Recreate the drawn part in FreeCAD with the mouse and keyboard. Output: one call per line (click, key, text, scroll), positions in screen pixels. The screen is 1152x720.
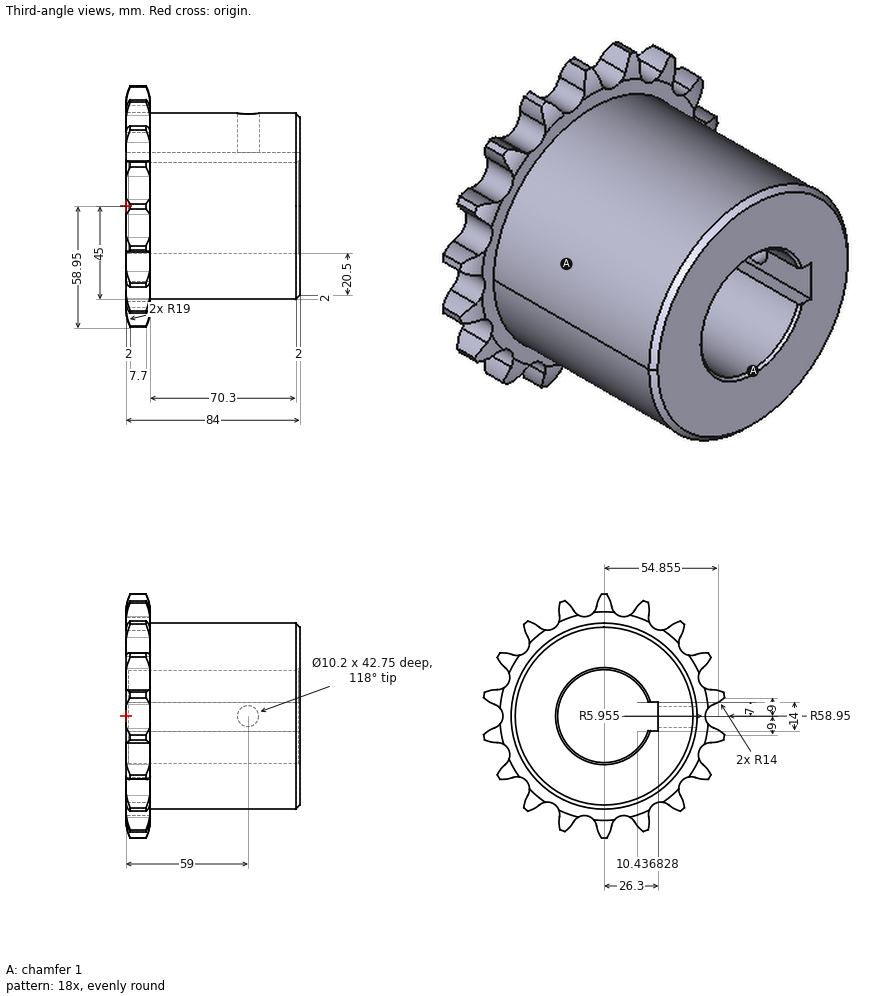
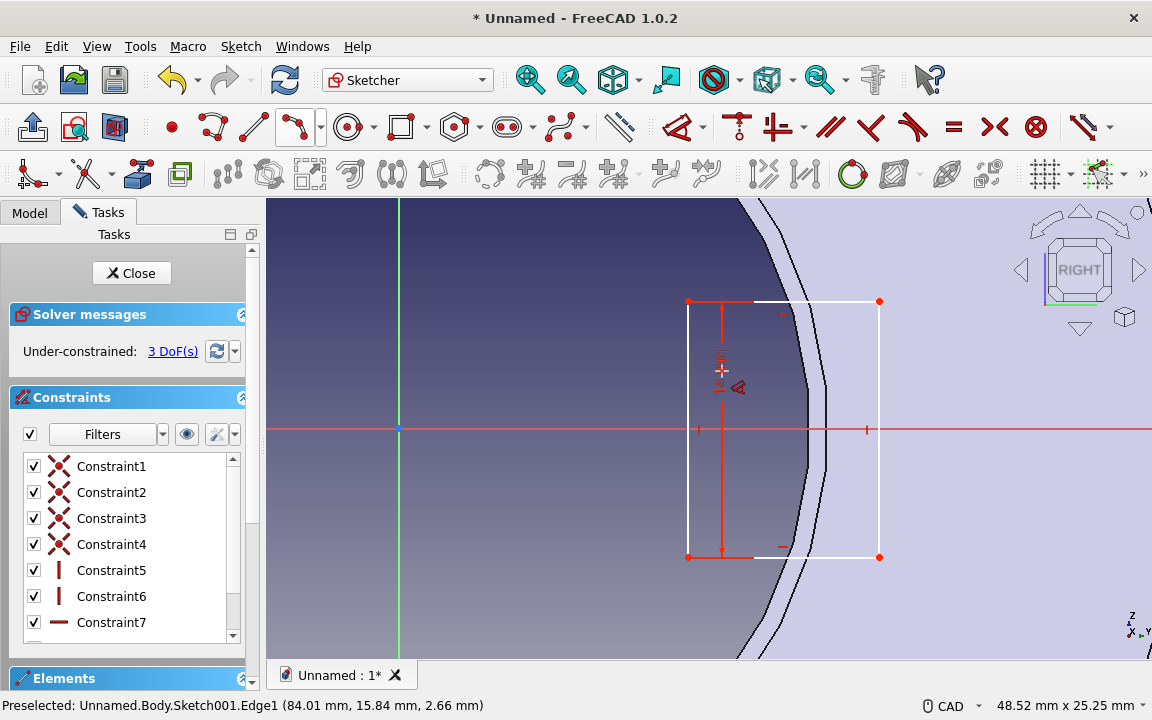
click(688, 302)
click(365, 365)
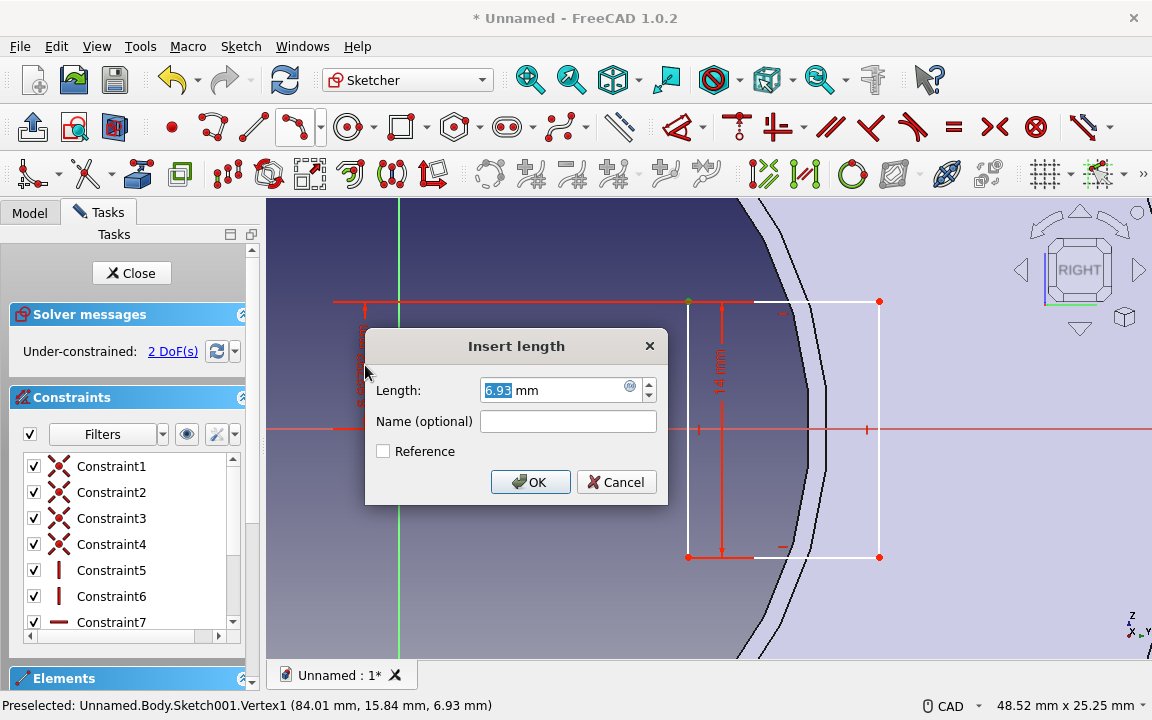
text(7)
key(Return)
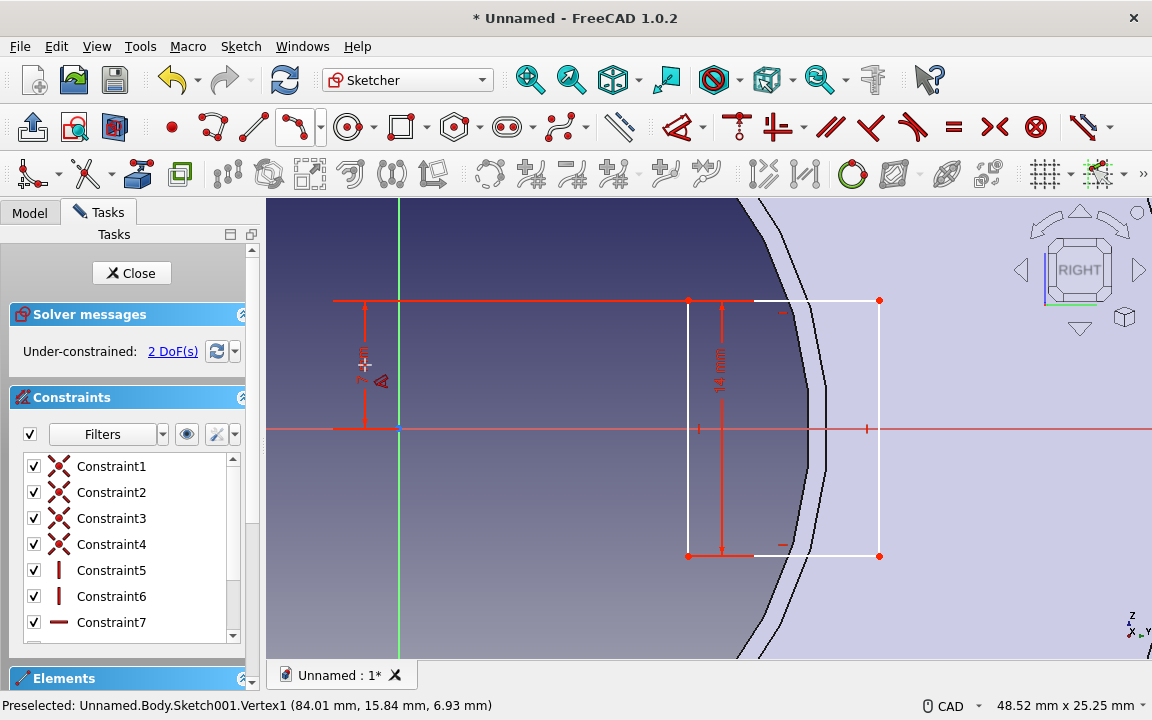
click(879, 556)
click(639, 590)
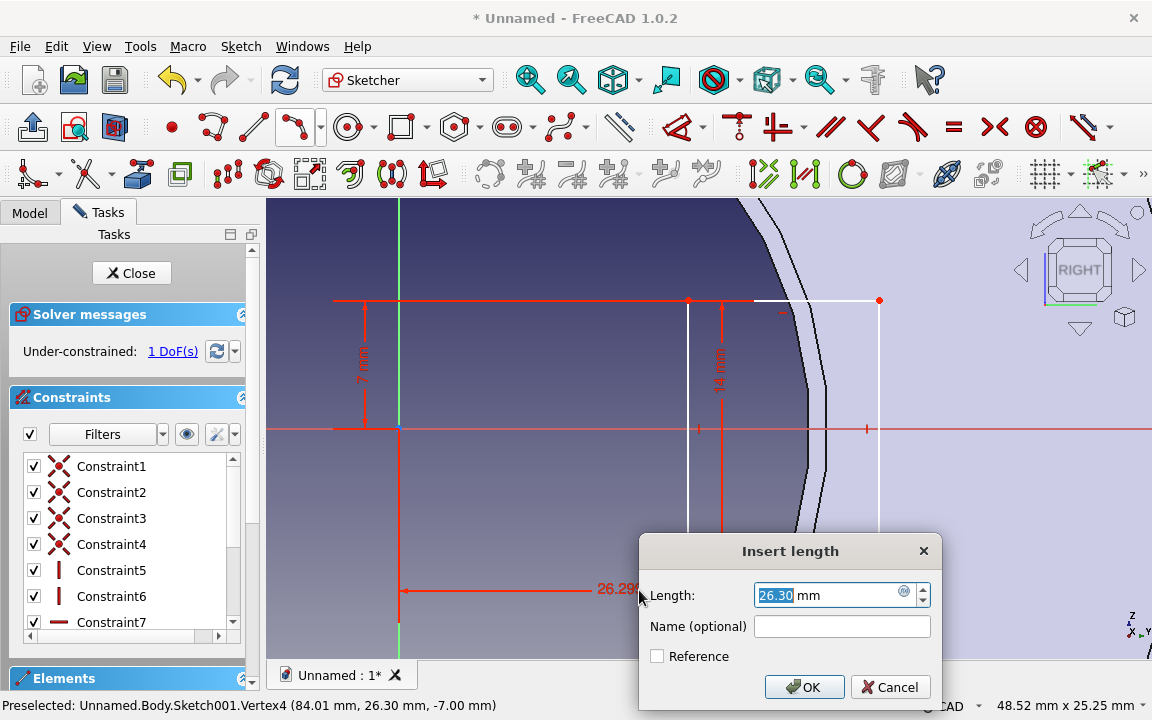
text(26.3)
key(Return)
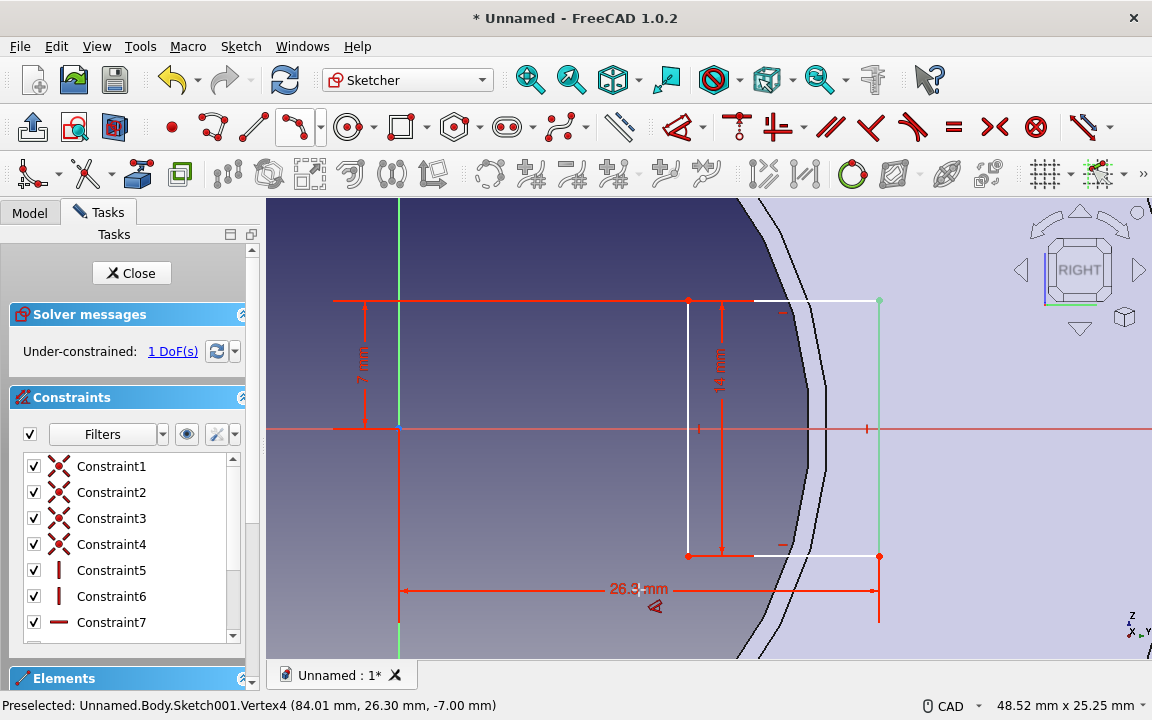
click(745, 556)
click(784, 590)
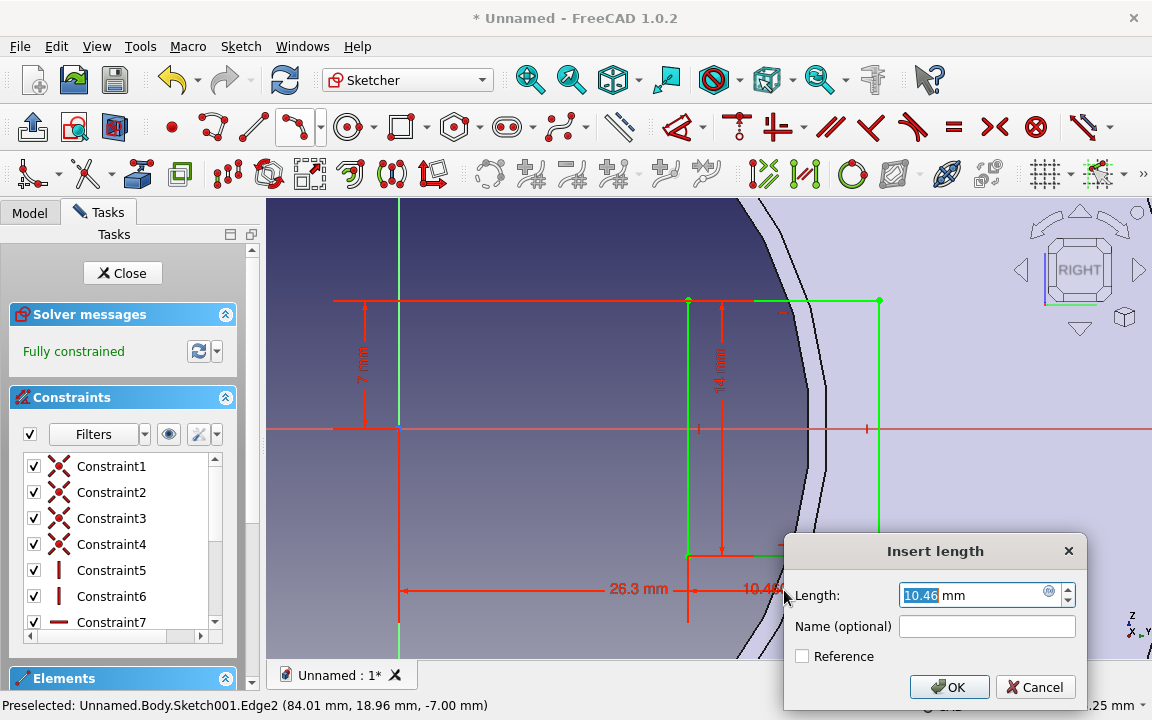
text(10.436828)
key(Return)
key(Escape)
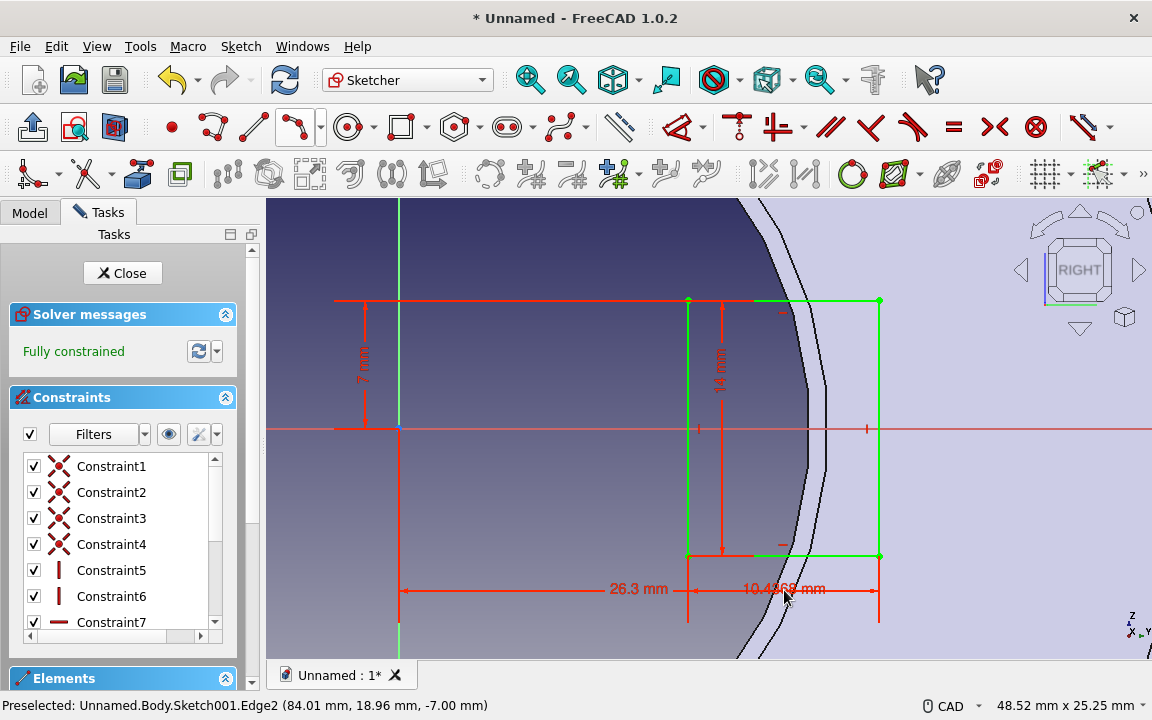
click(123, 273)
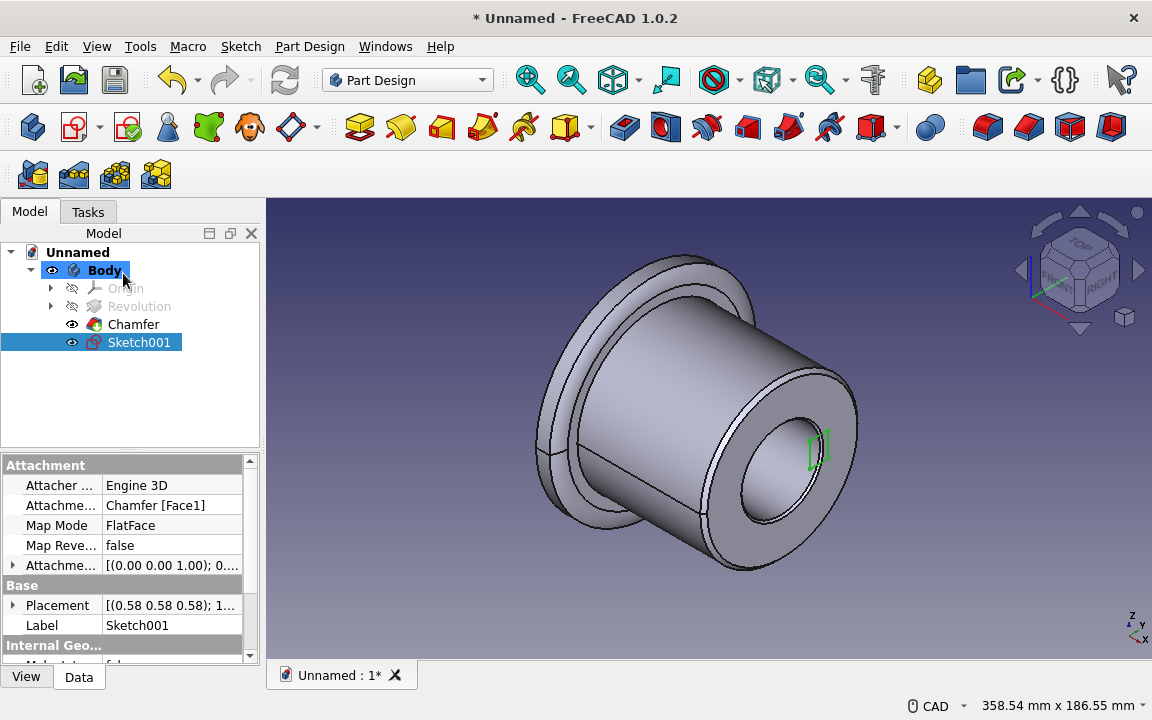
click(625, 128)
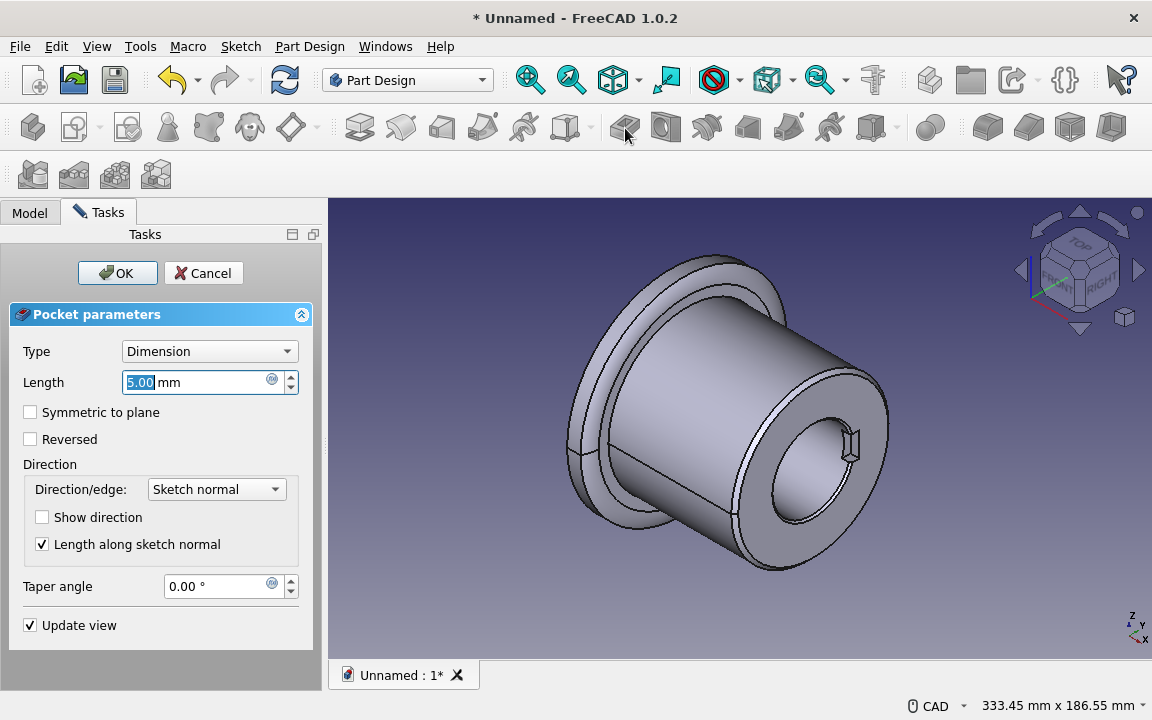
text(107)
key(Tab)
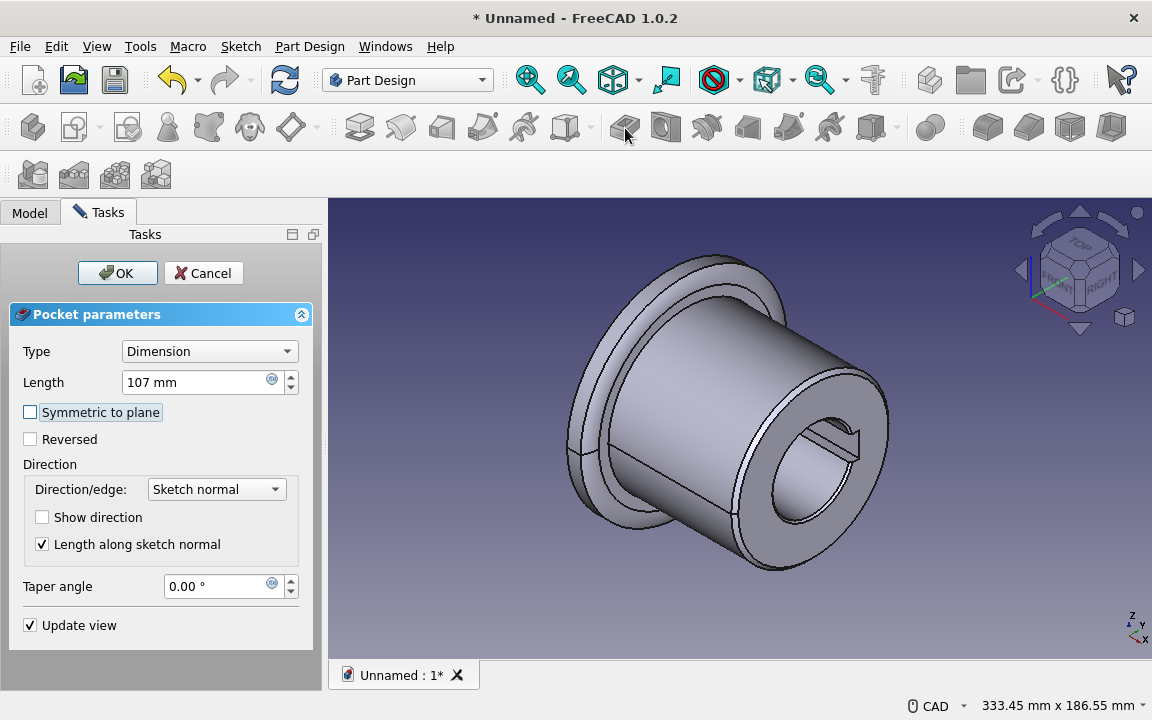
click(118, 273)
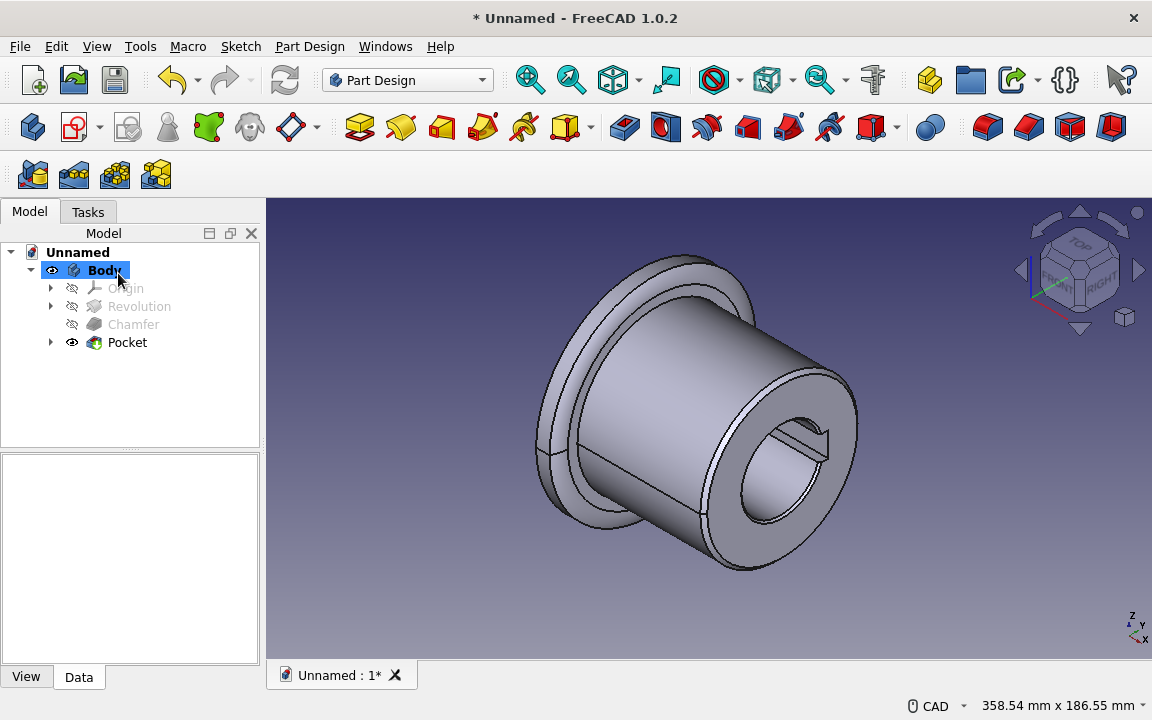
key(6)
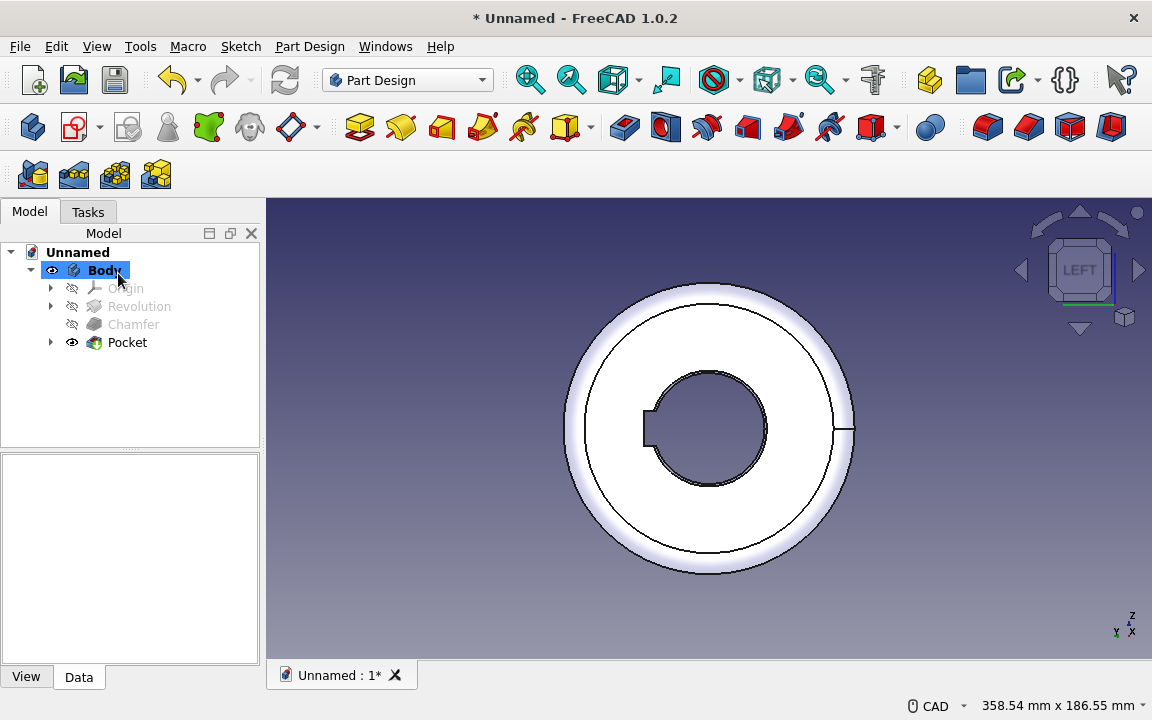
click(638, 499)